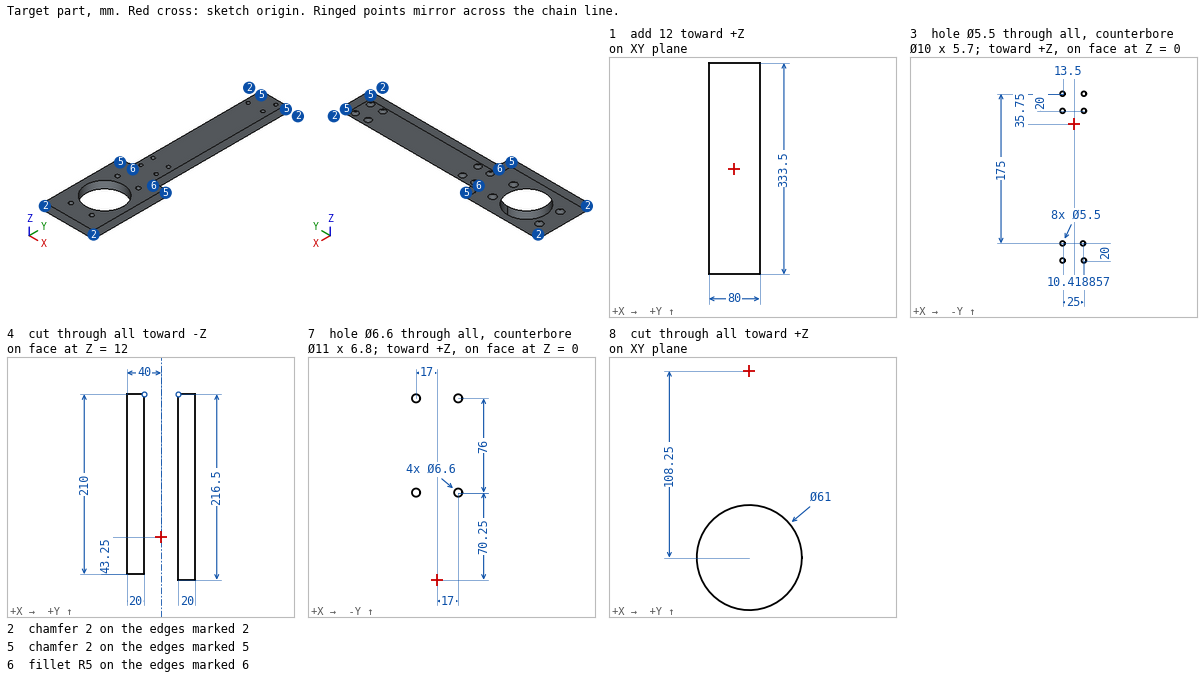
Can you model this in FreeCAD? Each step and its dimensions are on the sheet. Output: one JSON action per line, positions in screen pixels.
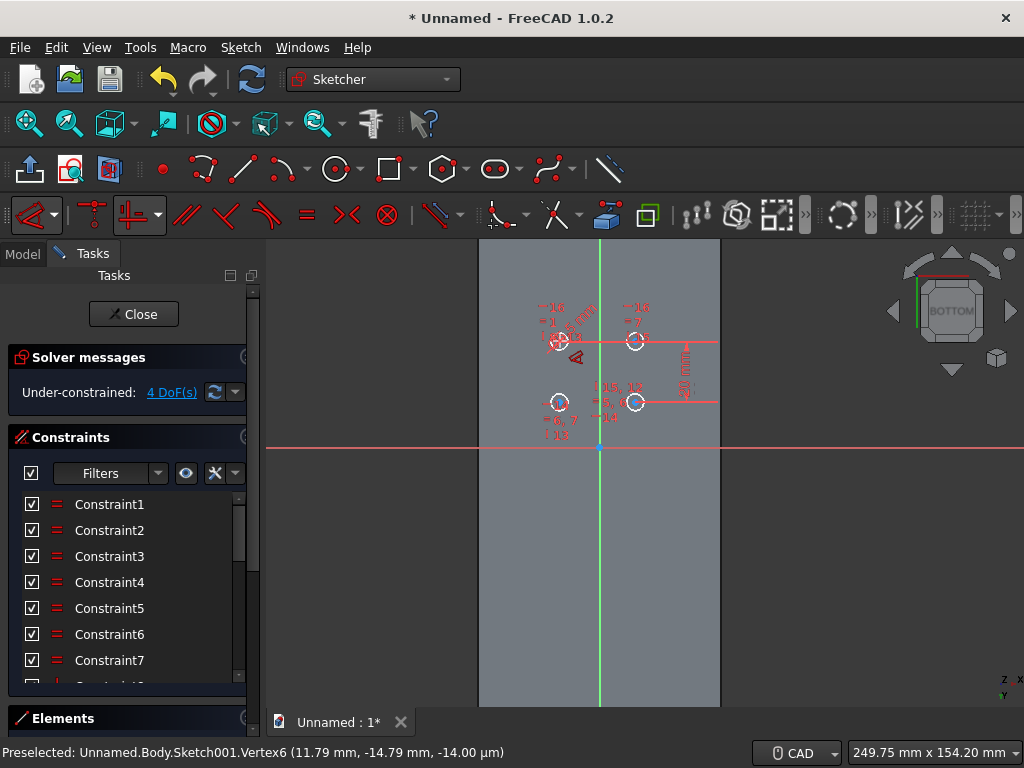
{"action": "left_click", "coordinate": [559, 342]}
{"action": "left_click", "coordinate": [579, 482]}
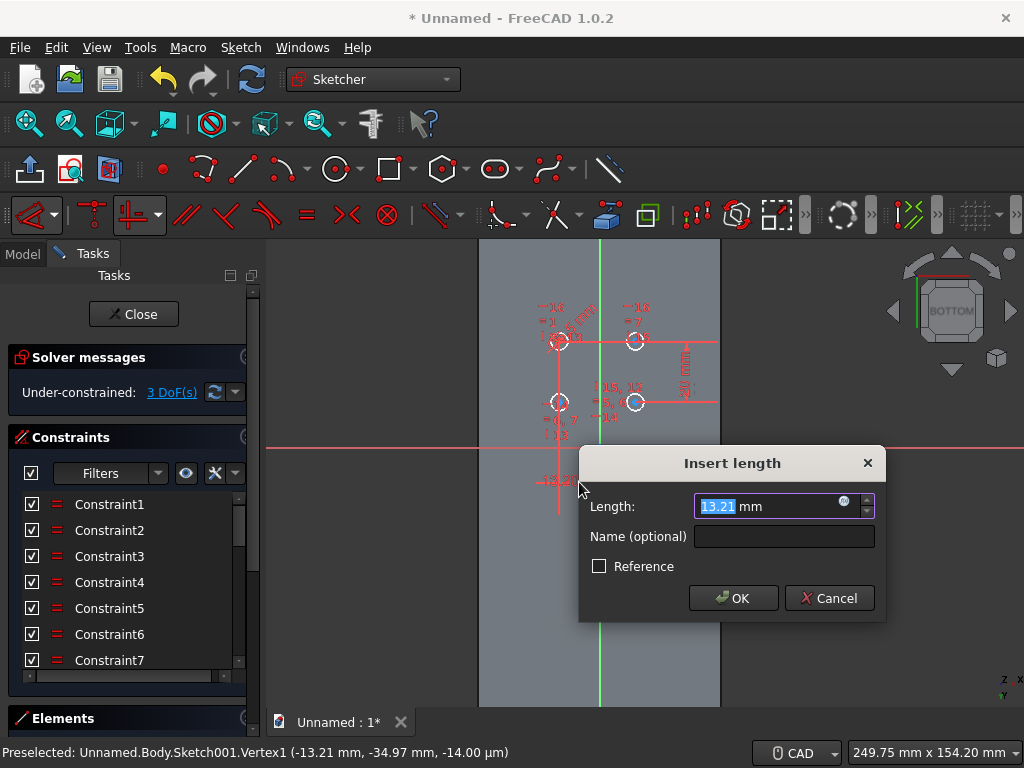
{"action": "type", "text": "13.5"}
{"action": "key", "text": "Return"}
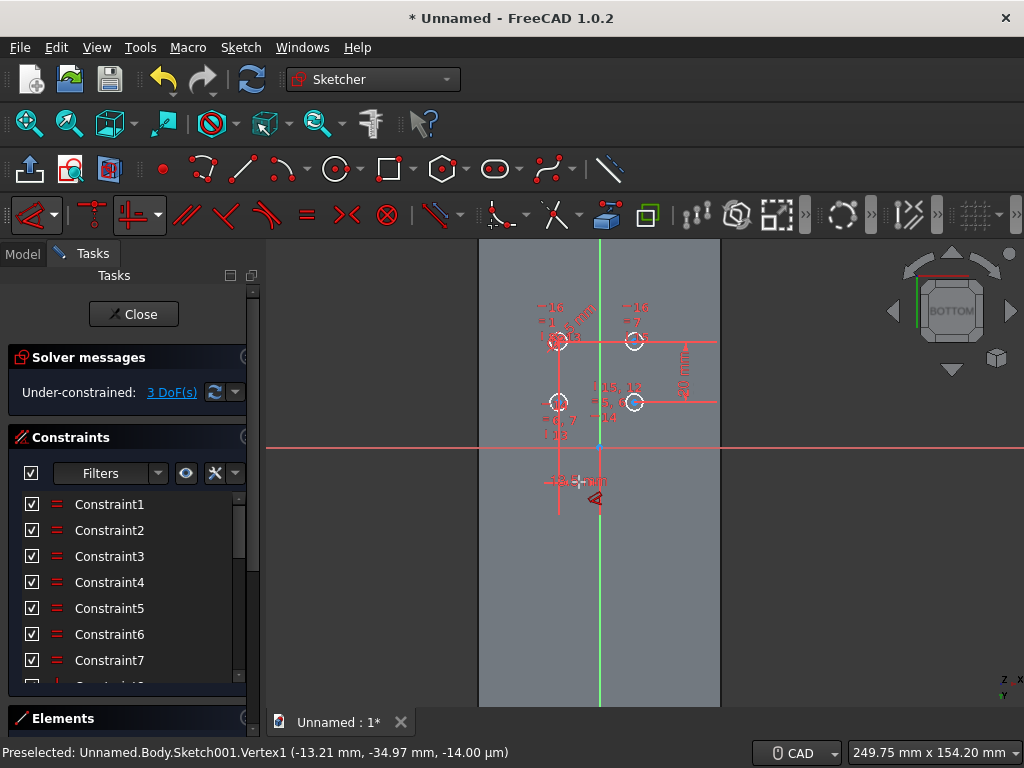
{"action": "left_click", "coordinate": [559, 342]}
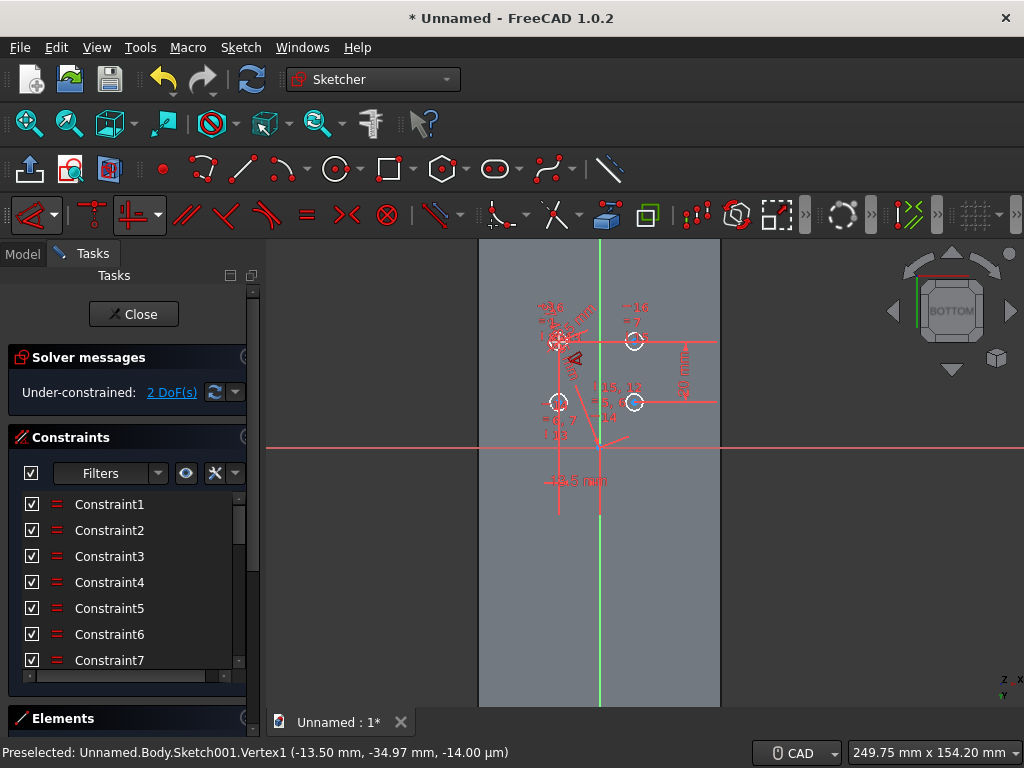
{"action": "scroll", "coordinate": [560, 341], "scroll_direction": "down", "scroll_amount": 4}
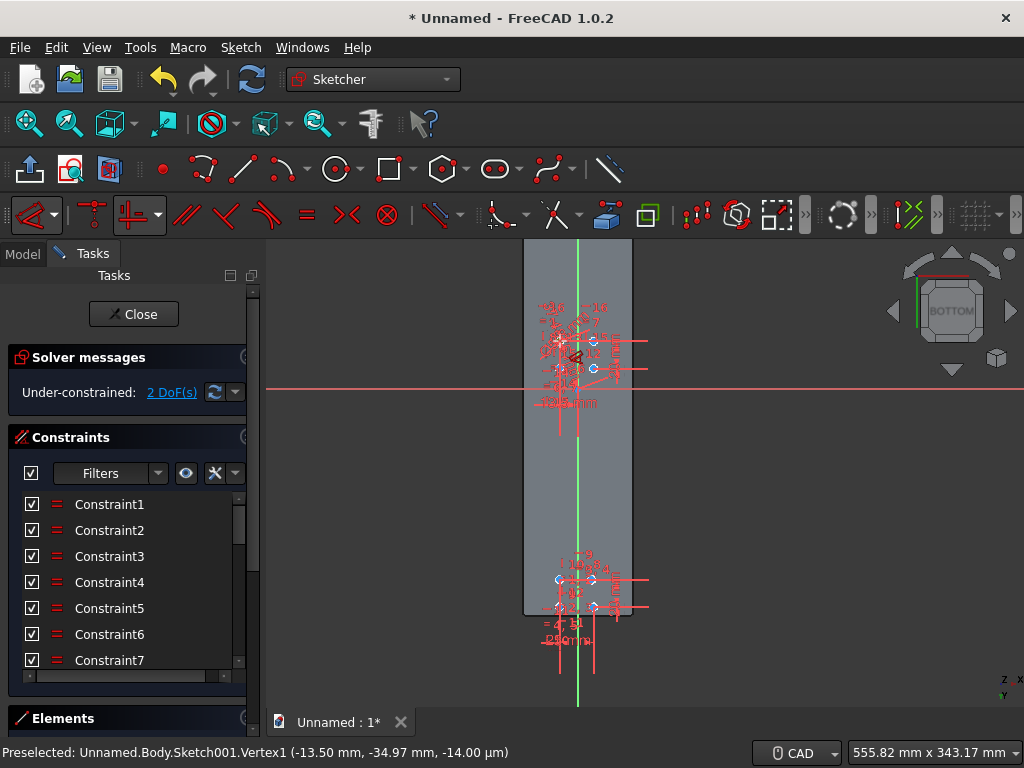
{"action": "left_click", "coordinate": [560, 580]}
{"action": "left_click", "coordinate": [526, 461]}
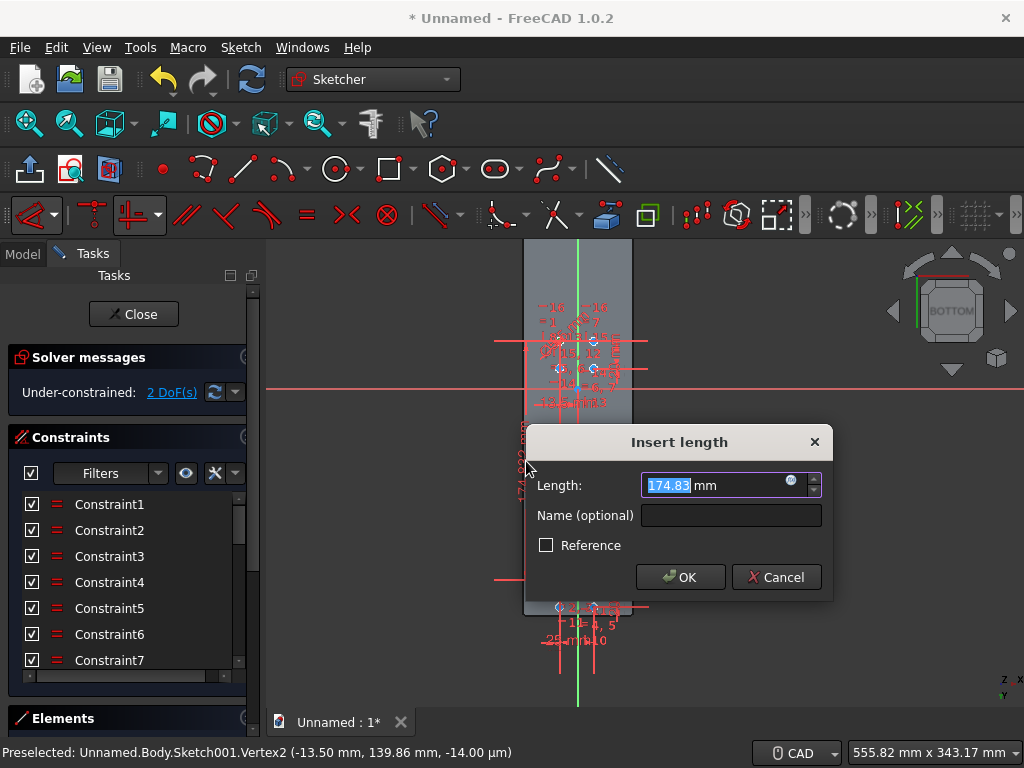
{"action": "type", "text": "175"}
{"action": "key", "text": "Return"}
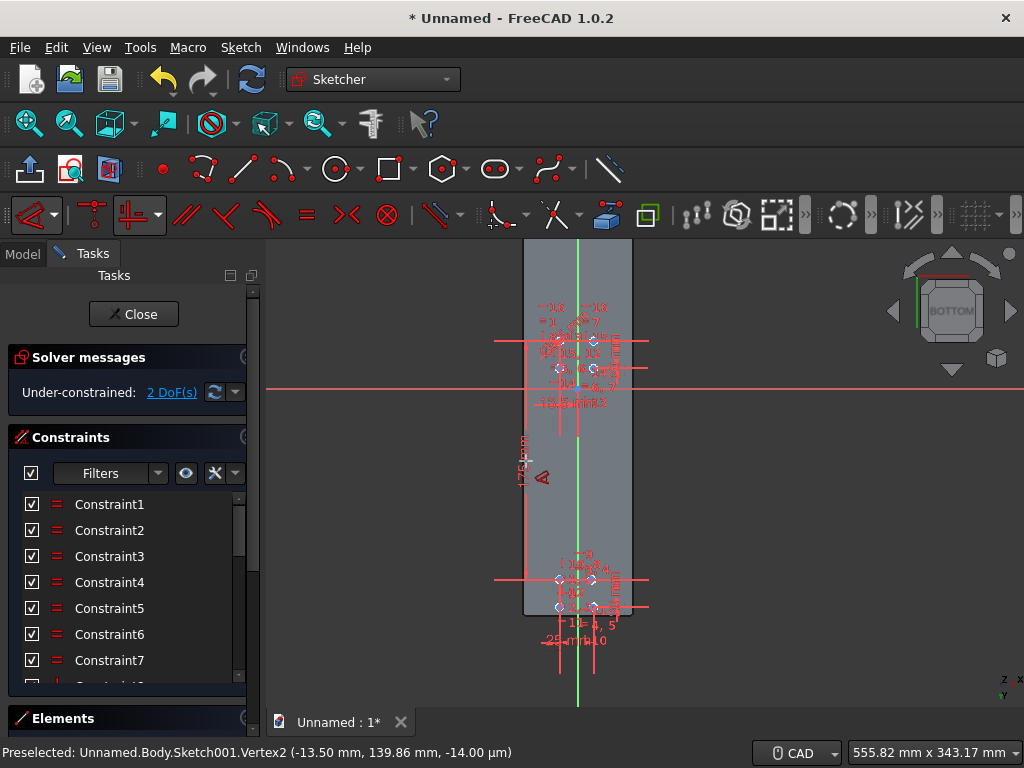
{"action": "left_click", "coordinate": [560, 341]}
{"action": "left_click", "coordinate": [526, 365]}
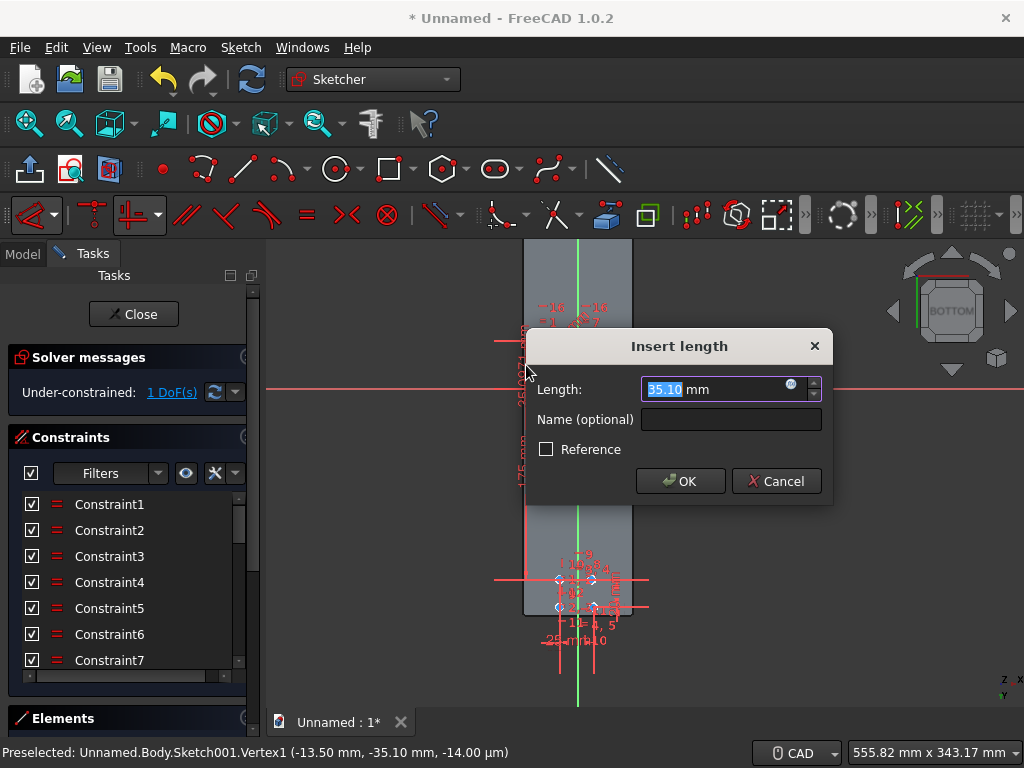
{"action": "type", "text": "35.75"}
{"action": "key", "text": "Return"}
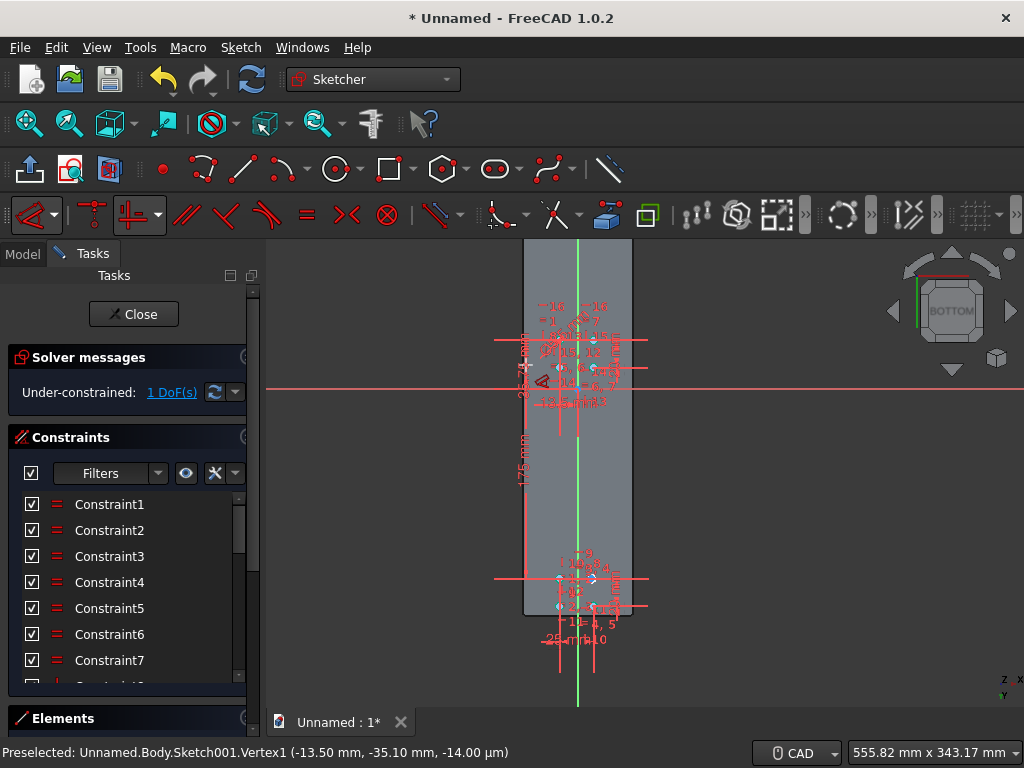
{"action": "scroll", "coordinate": [592, 579], "scroll_direction": "up", "scroll_amount": 6}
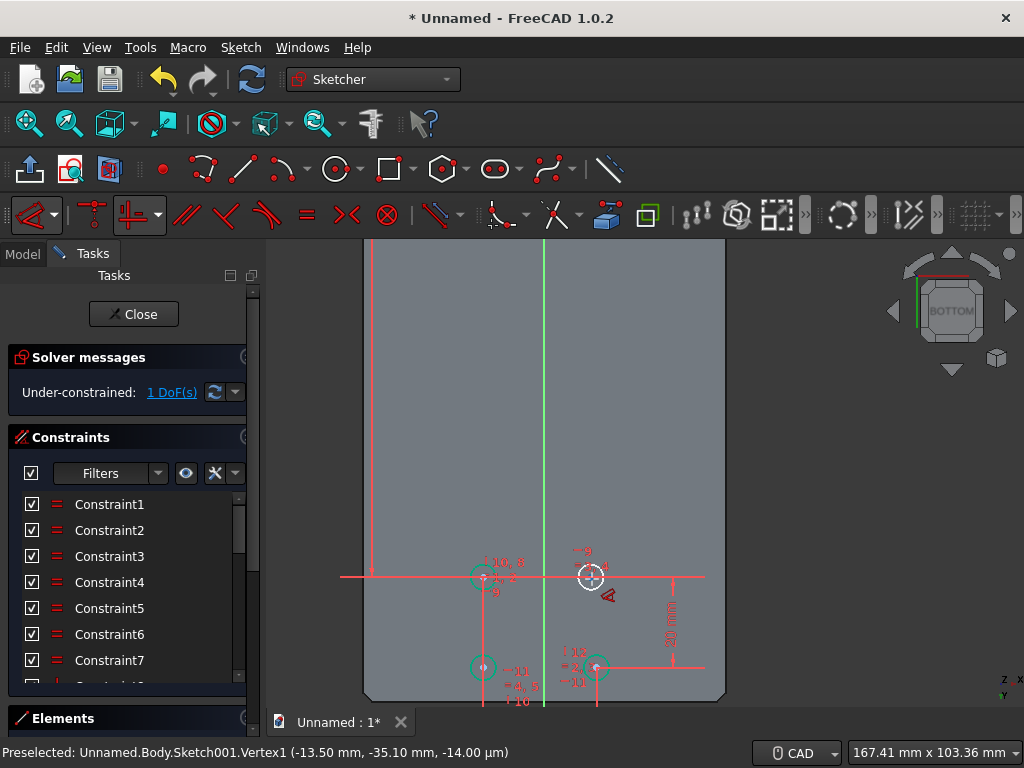
{"action": "left_click", "coordinate": [591, 577]}
{"action": "left_click", "coordinate": [568, 611]}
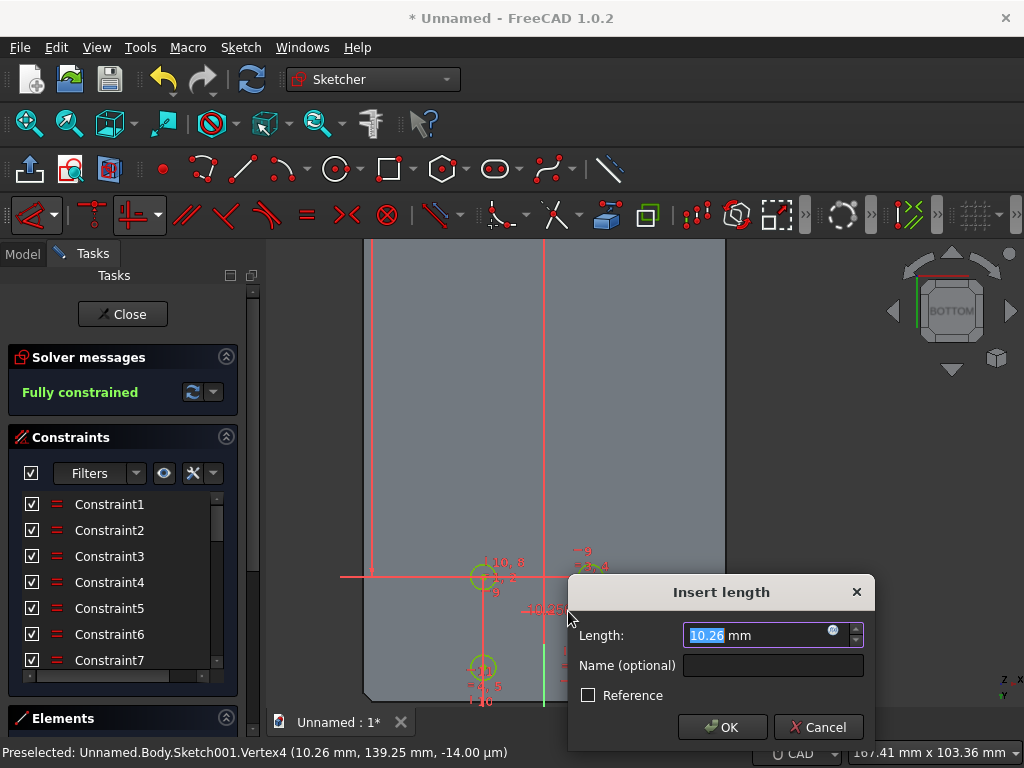
{"action": "type", "text": "10.418857"}
{"action": "key", "text": "Return"}
{"action": "key", "text": "Escape"}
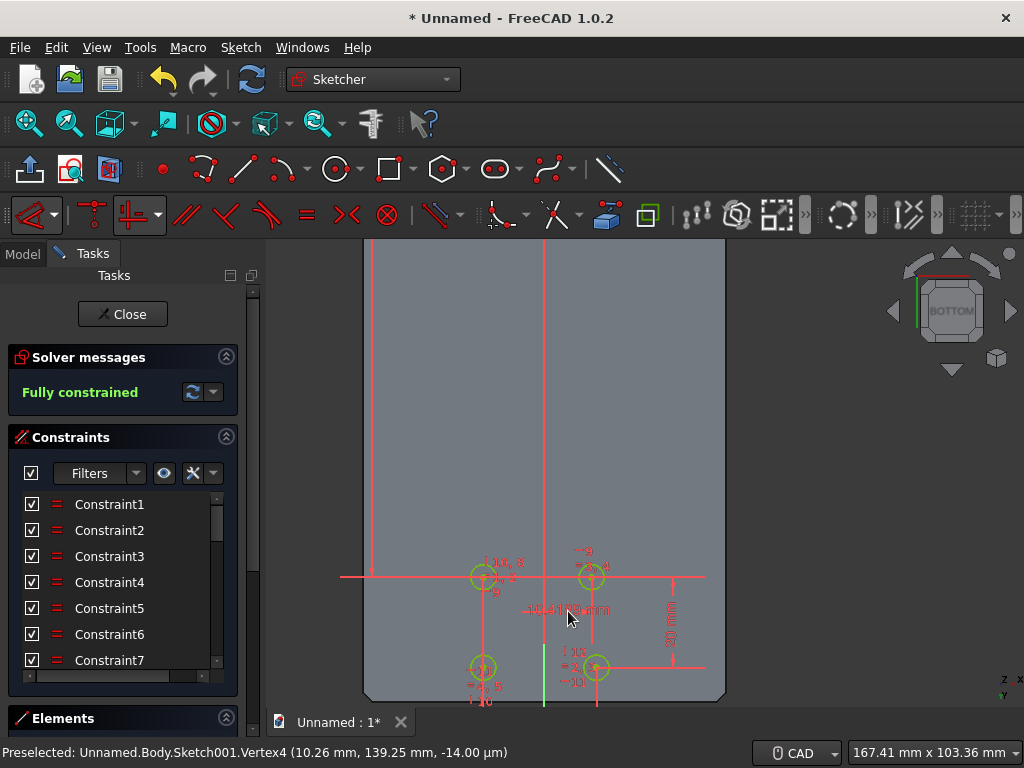
{"action": "left_click", "coordinate": [123, 314]}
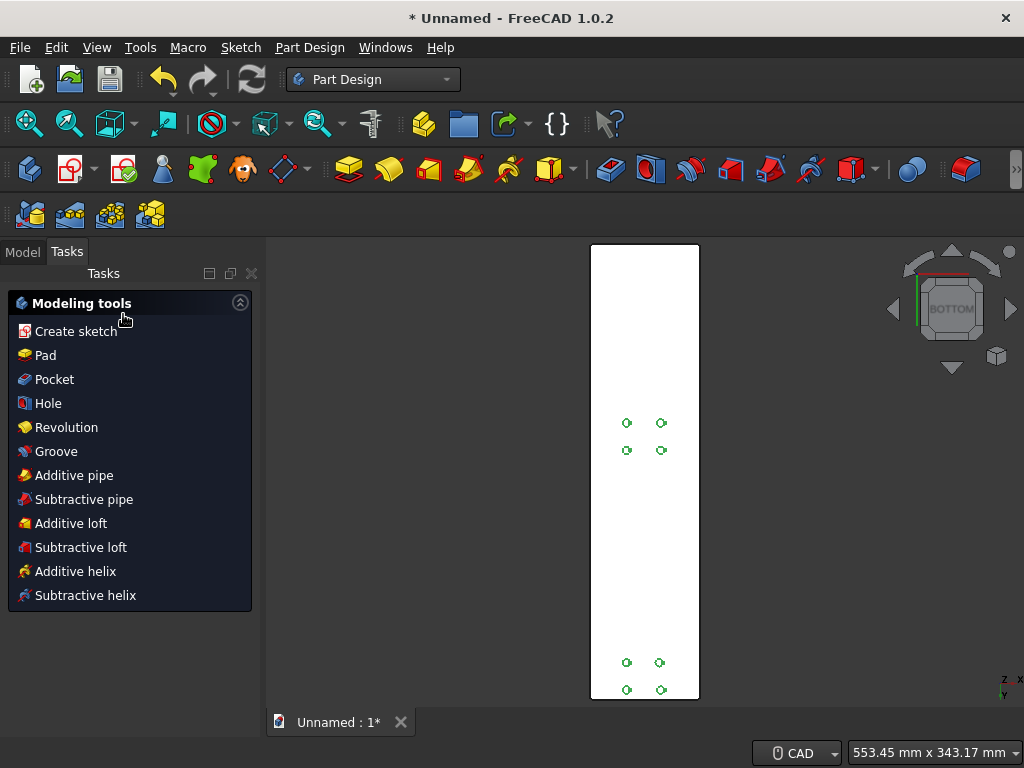
{"action": "left_click", "coordinate": [652, 170]}